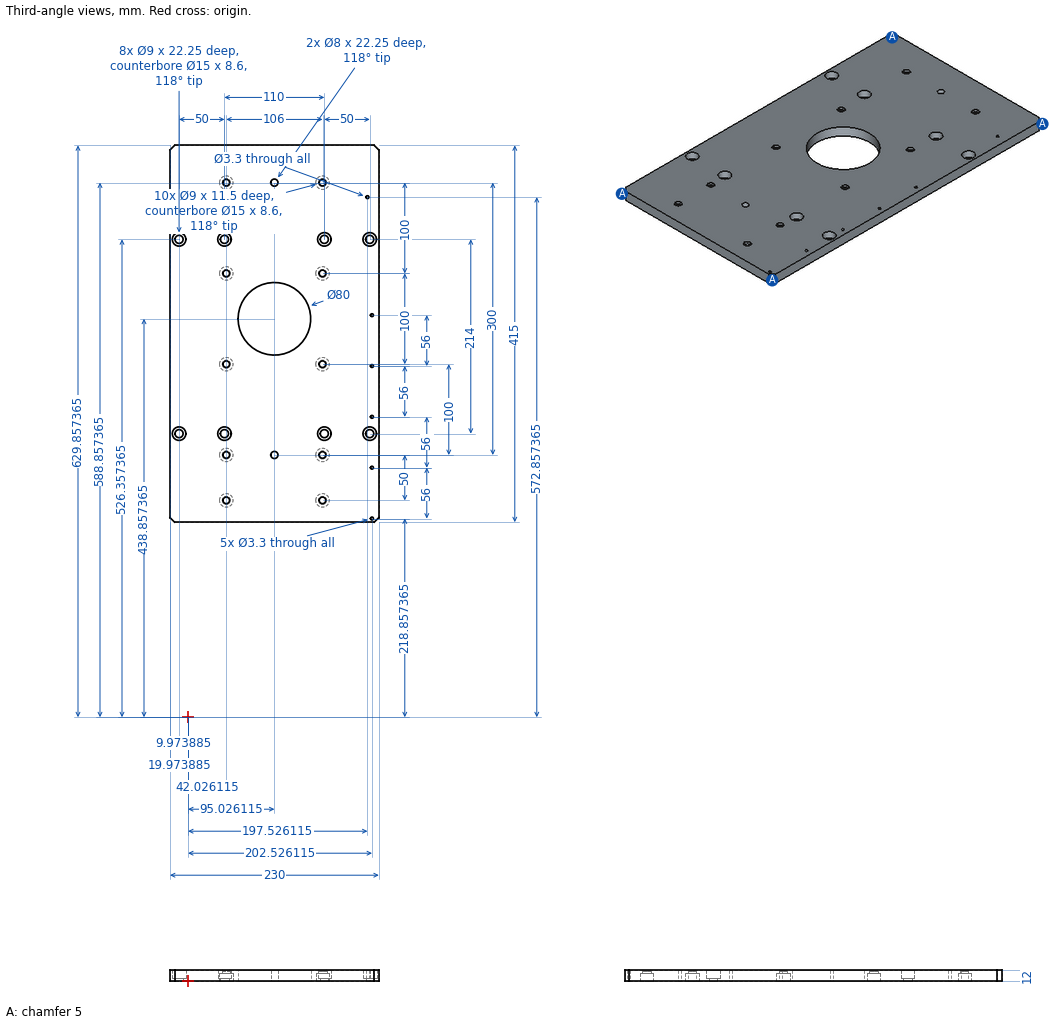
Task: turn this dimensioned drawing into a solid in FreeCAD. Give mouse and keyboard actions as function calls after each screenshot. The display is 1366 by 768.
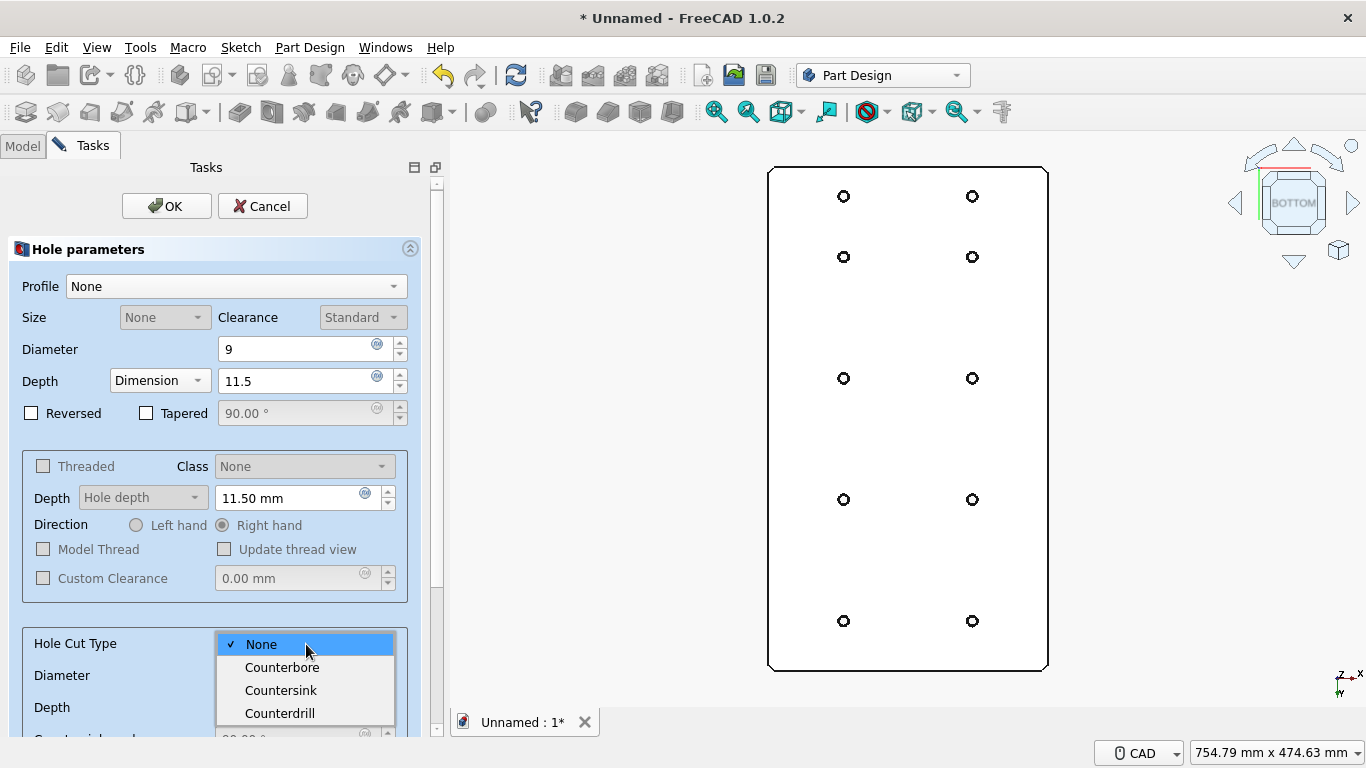
click(304, 668)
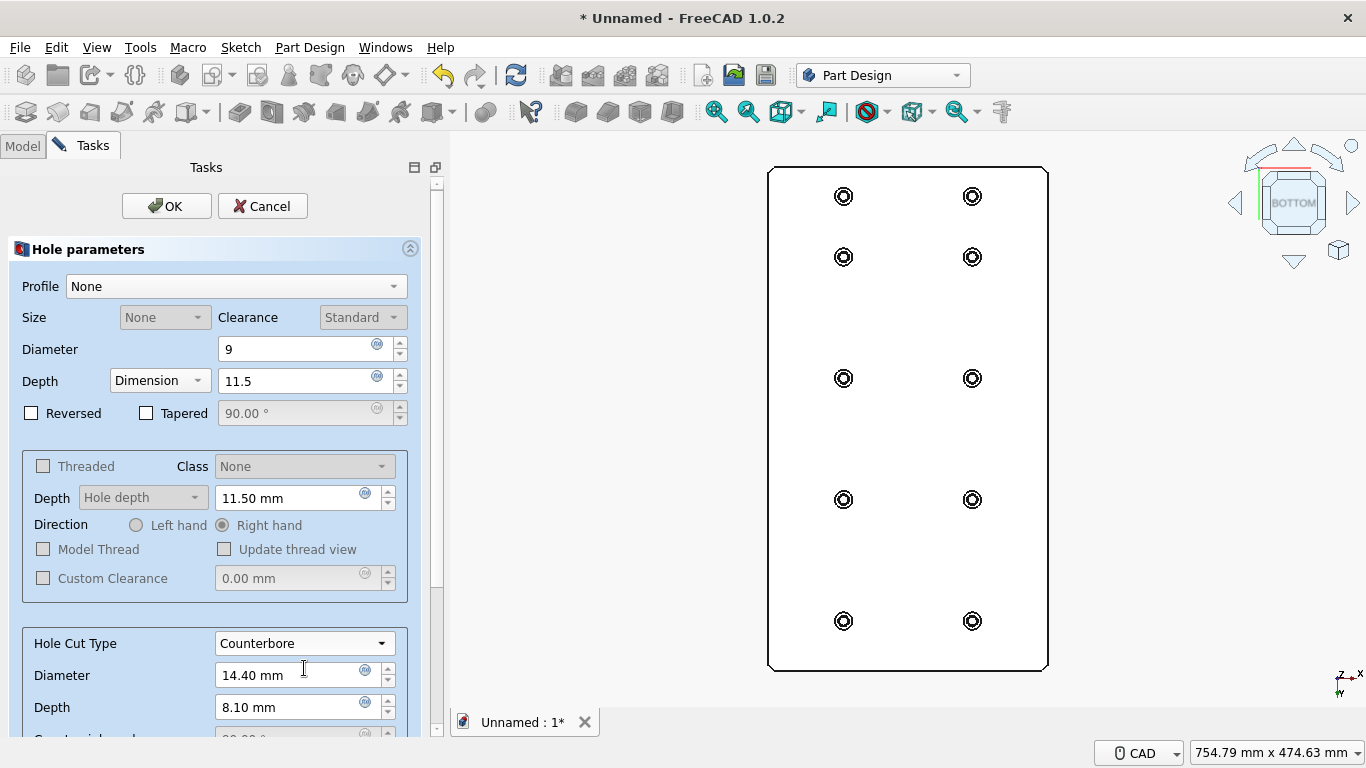
triple_click(298, 675)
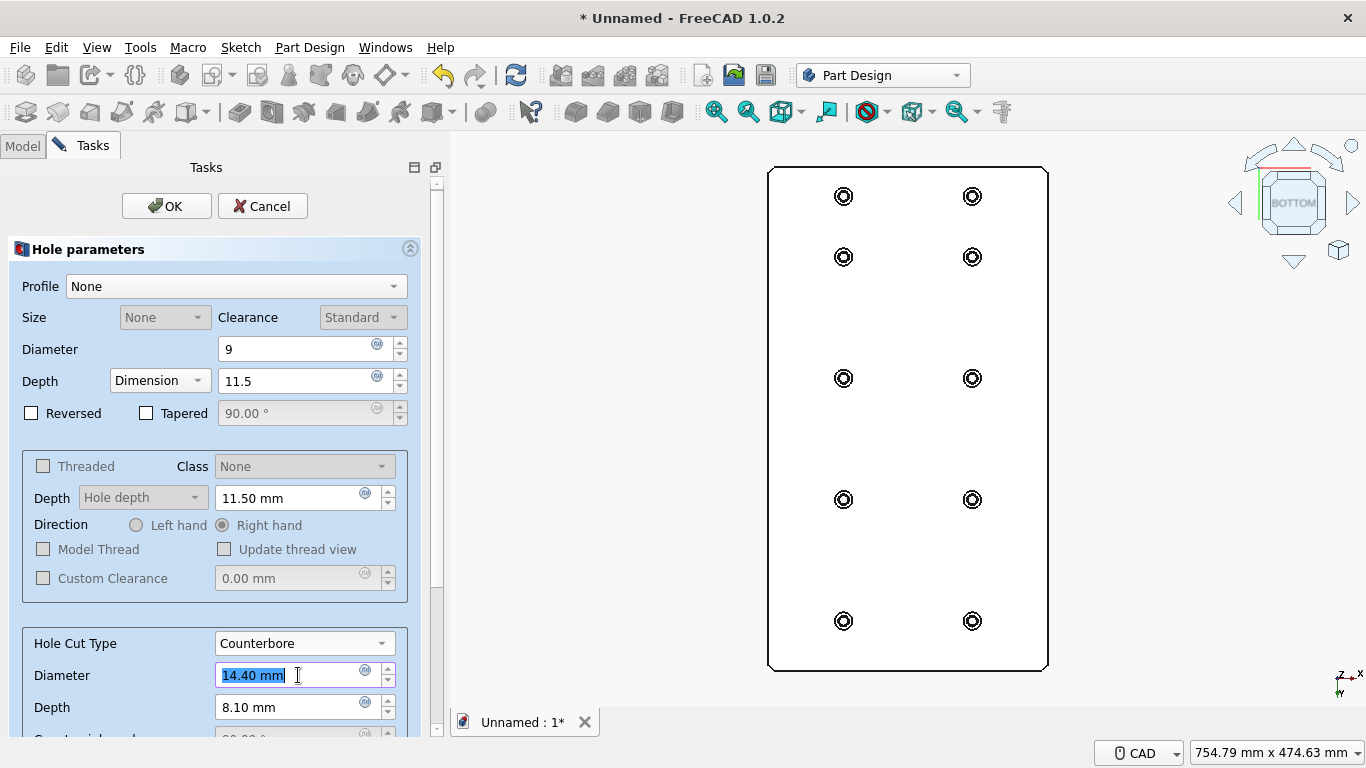
text(15)
key(Tab)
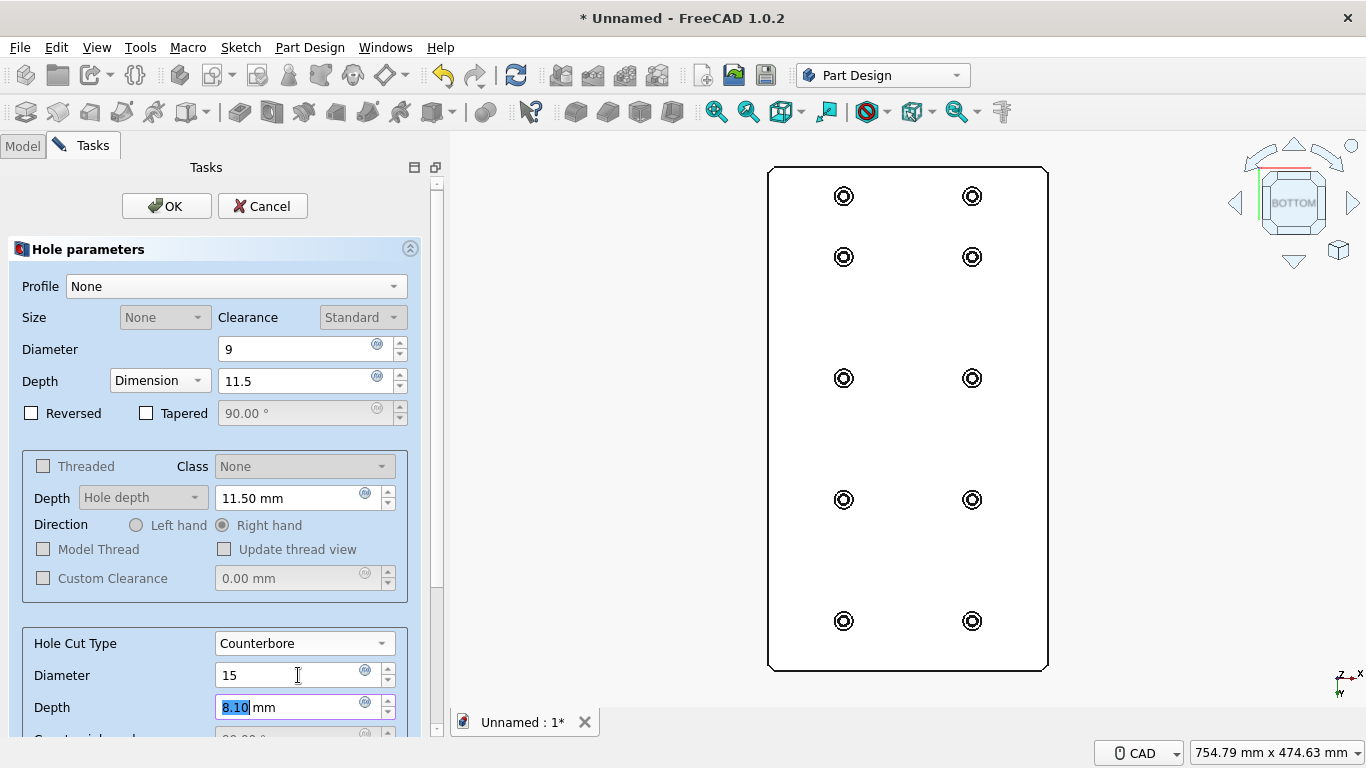
text(8.6)
key(Tab)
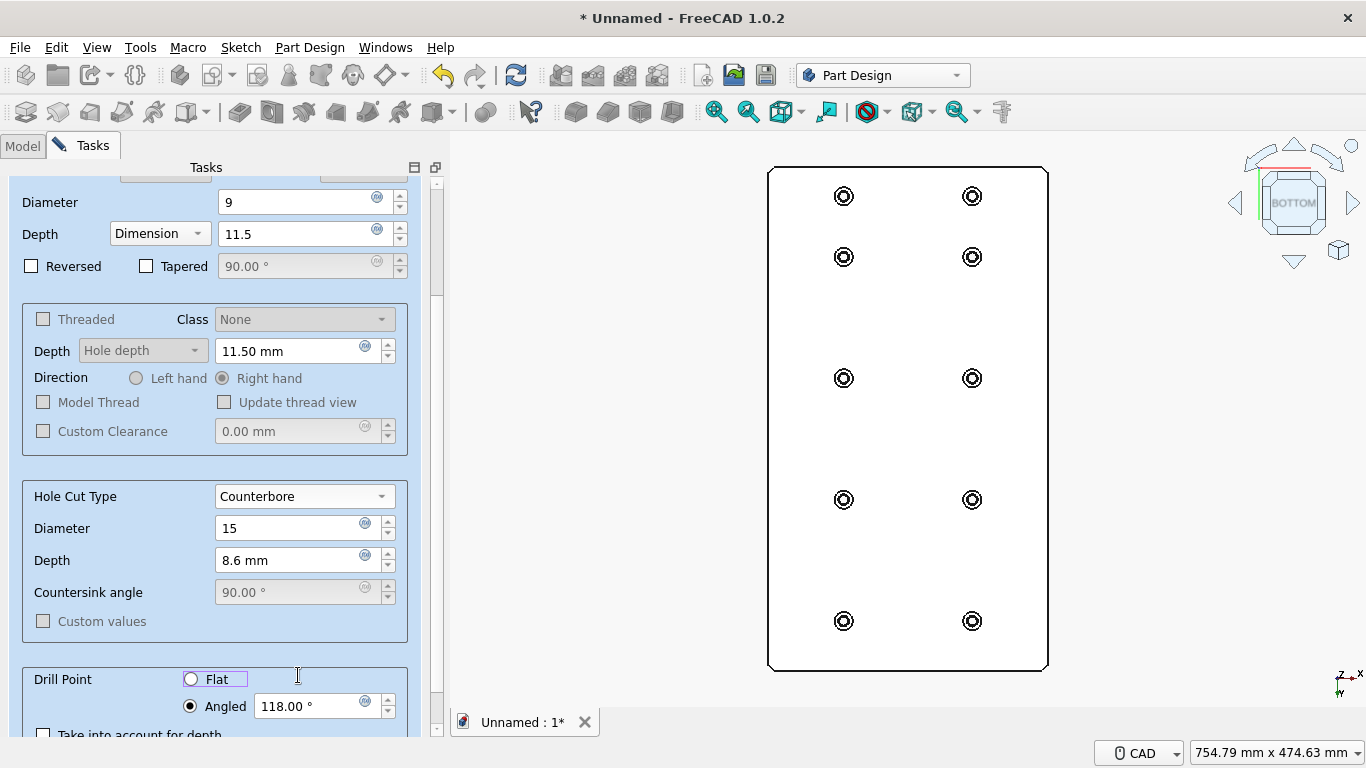
scroll(437, 456, up, 4)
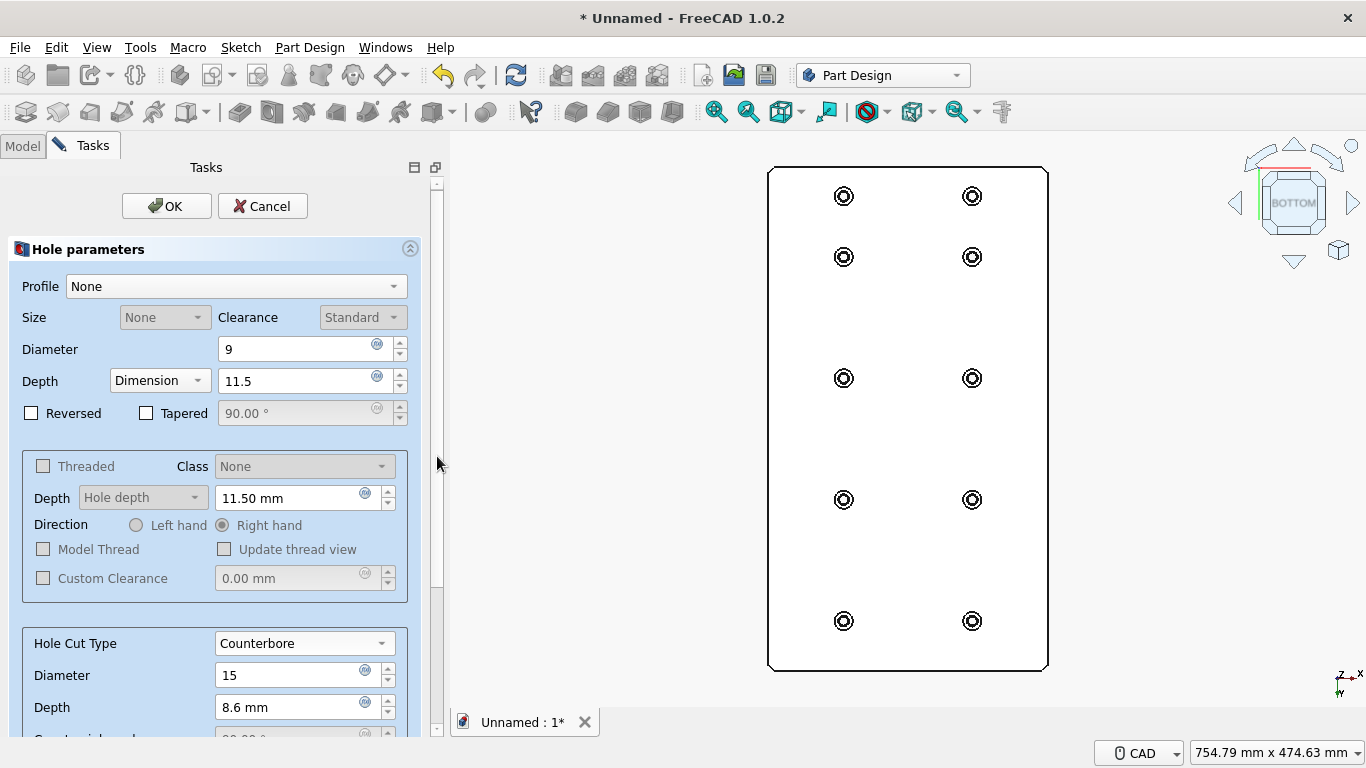
click(167, 206)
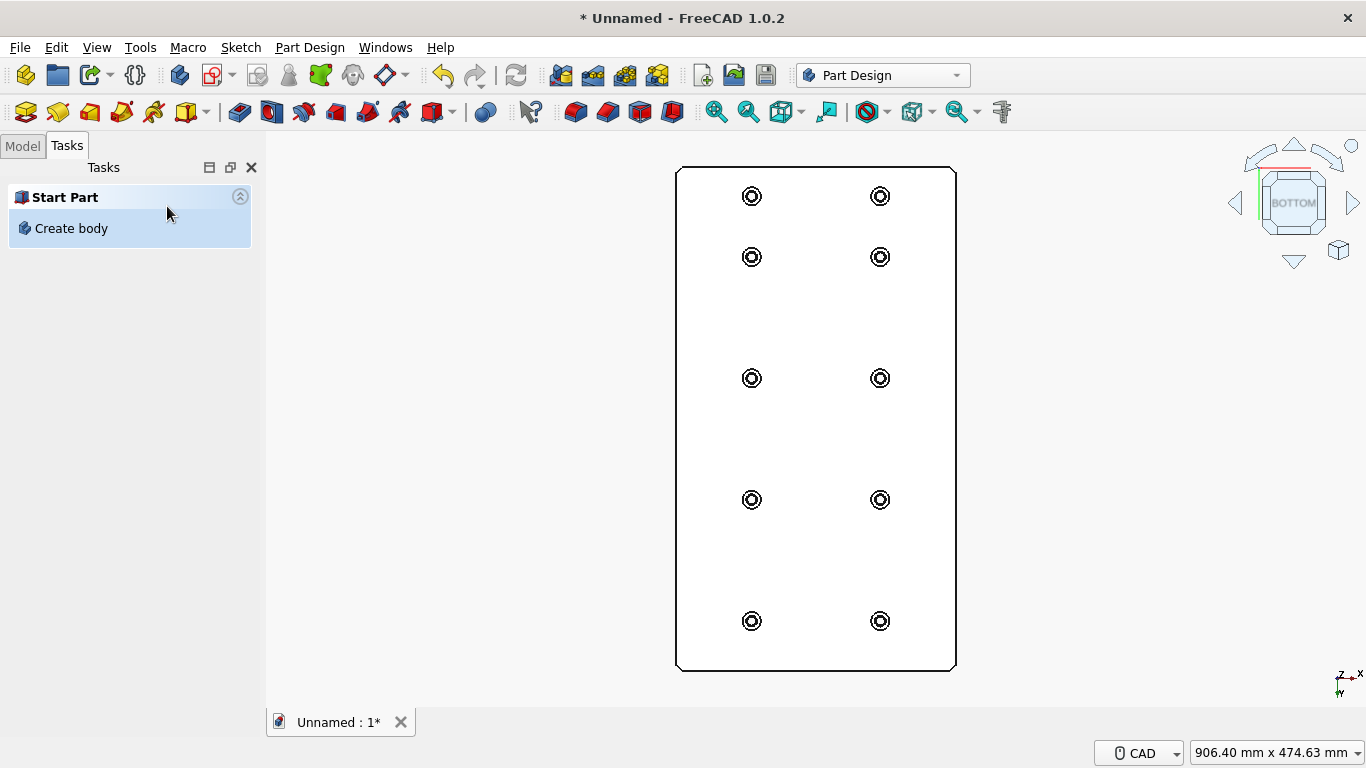
key(0)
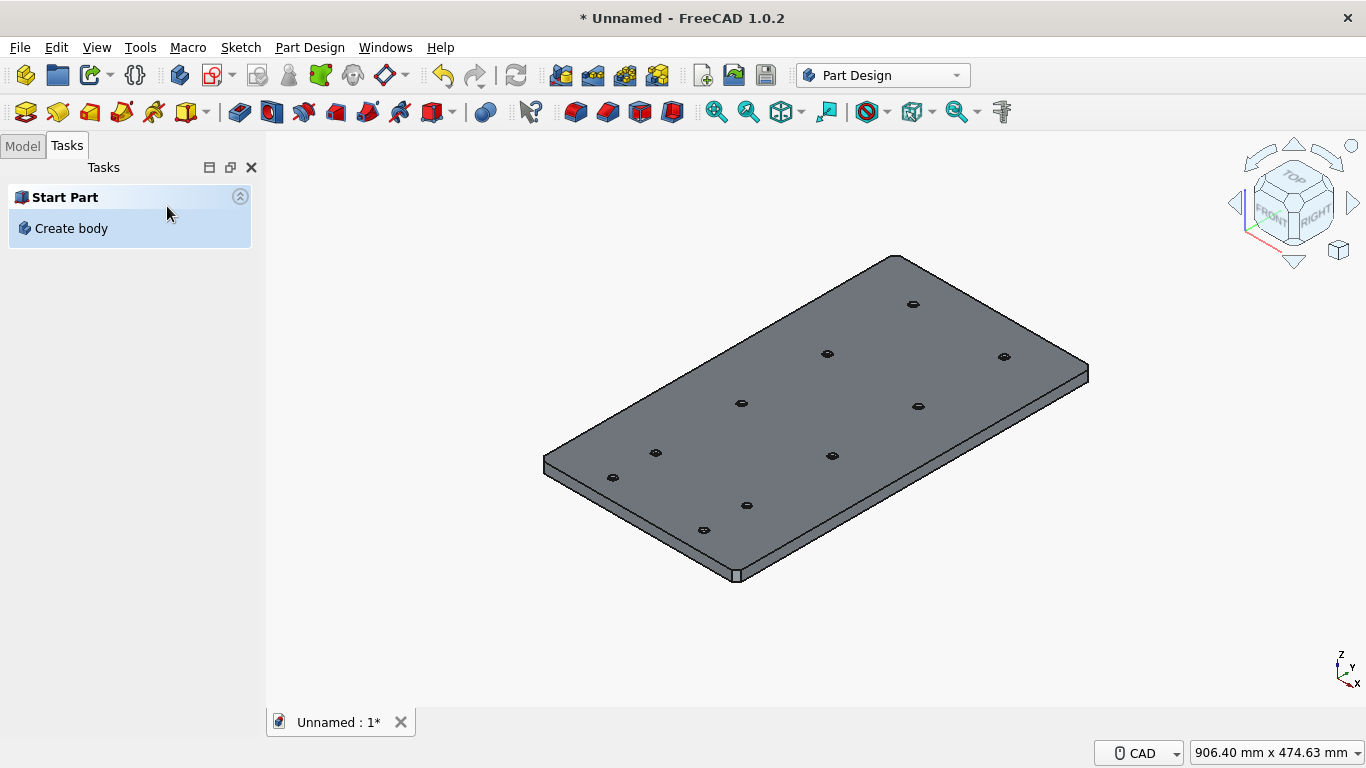
click(918, 353)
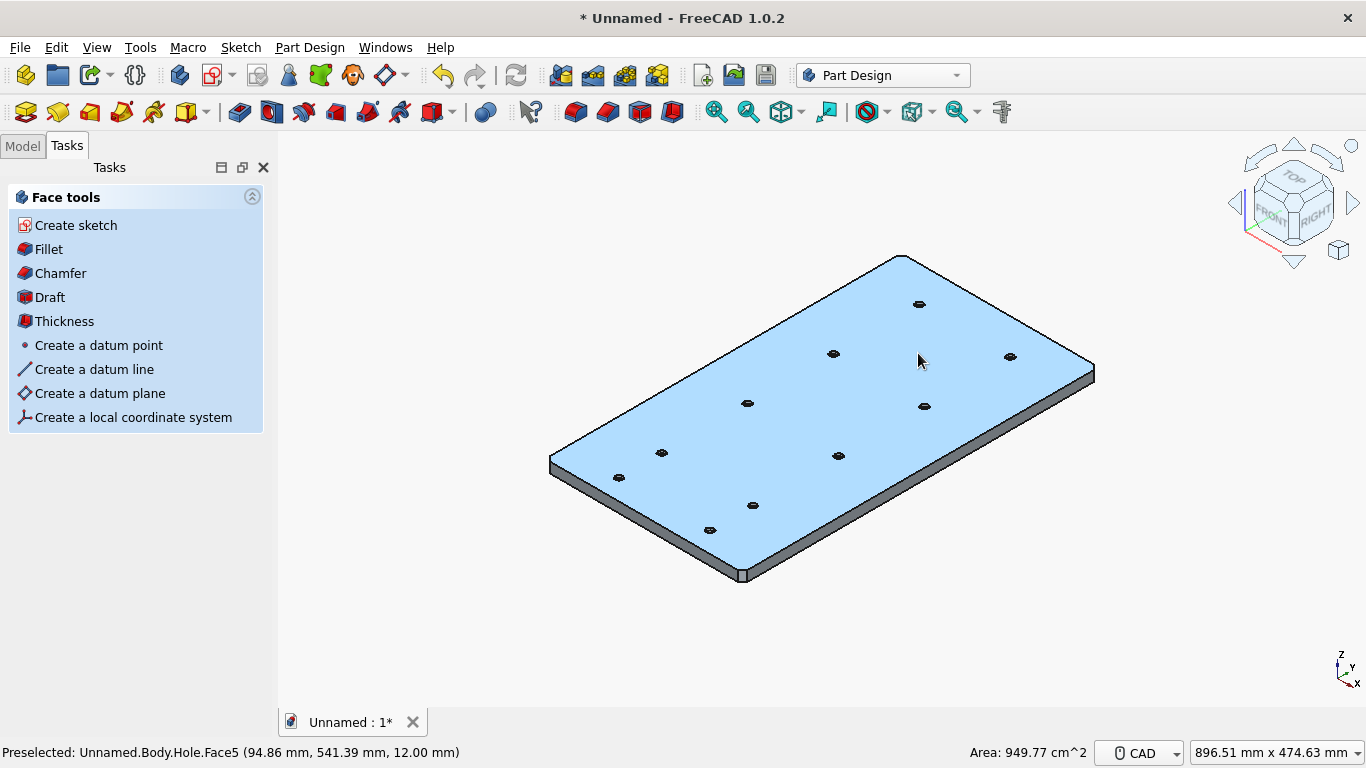
click(212, 76)